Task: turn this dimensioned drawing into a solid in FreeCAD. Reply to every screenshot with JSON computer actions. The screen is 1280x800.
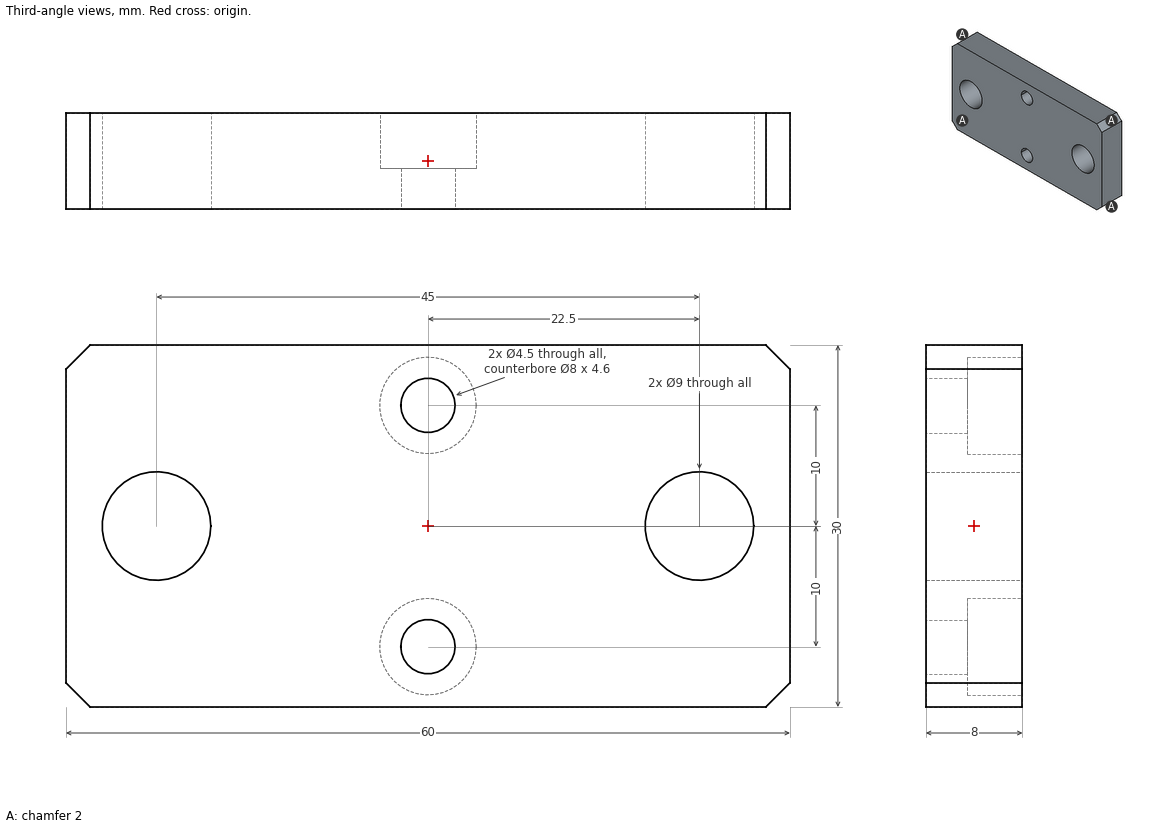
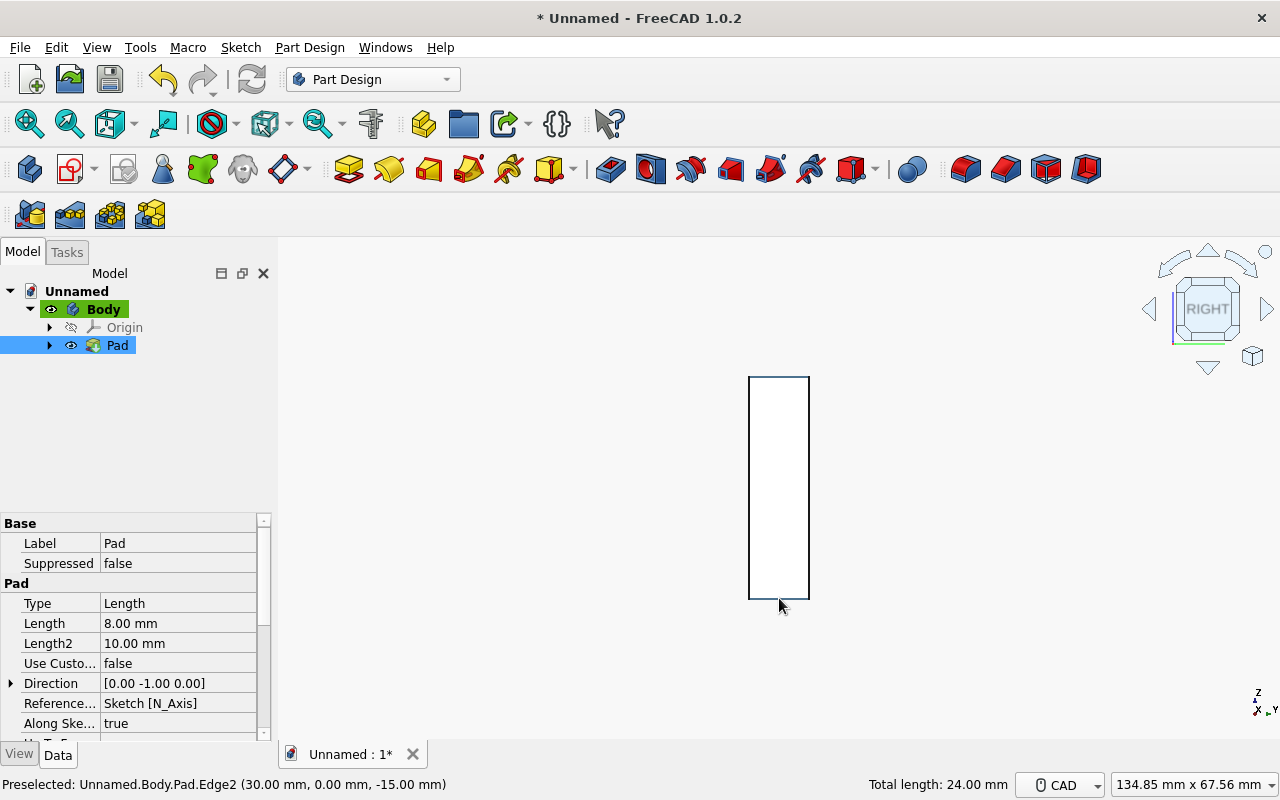
{"action": "key", "text": "5"}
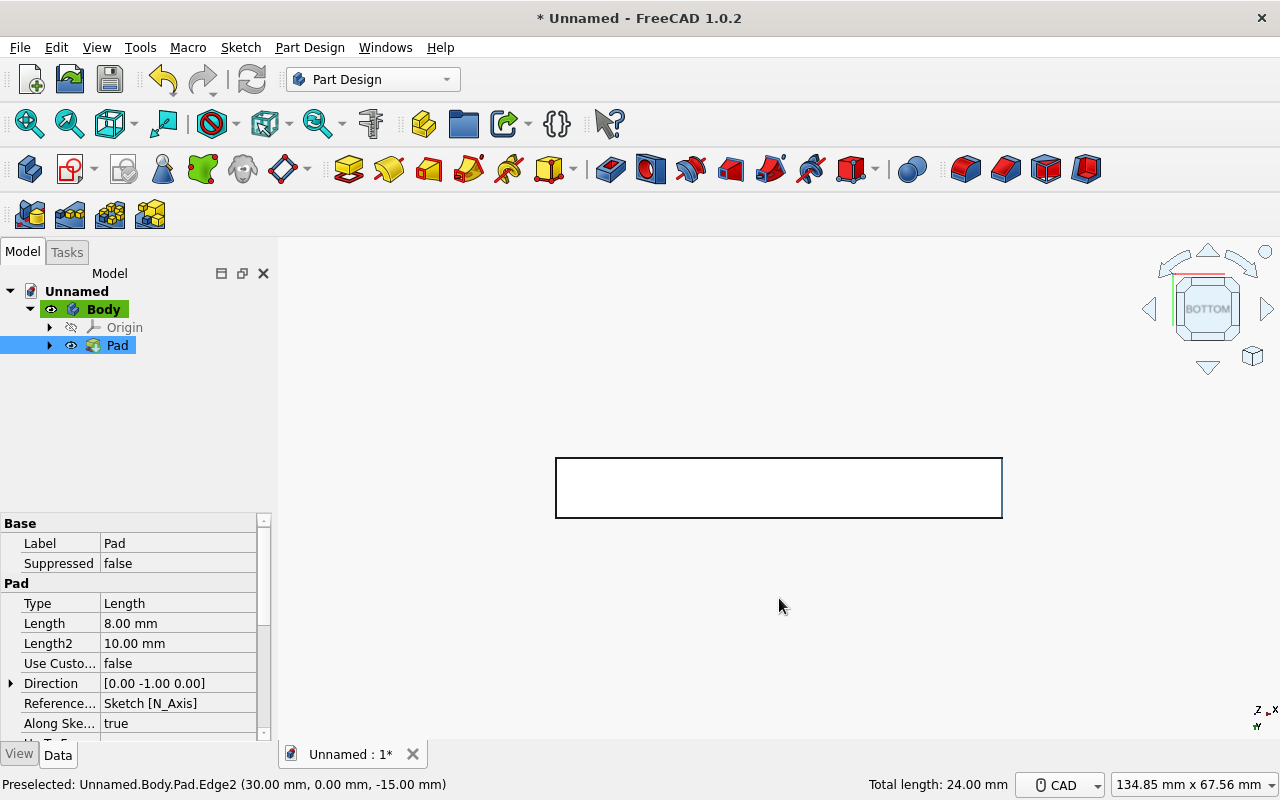
{"action": "left_click", "coordinate": [30, 124]}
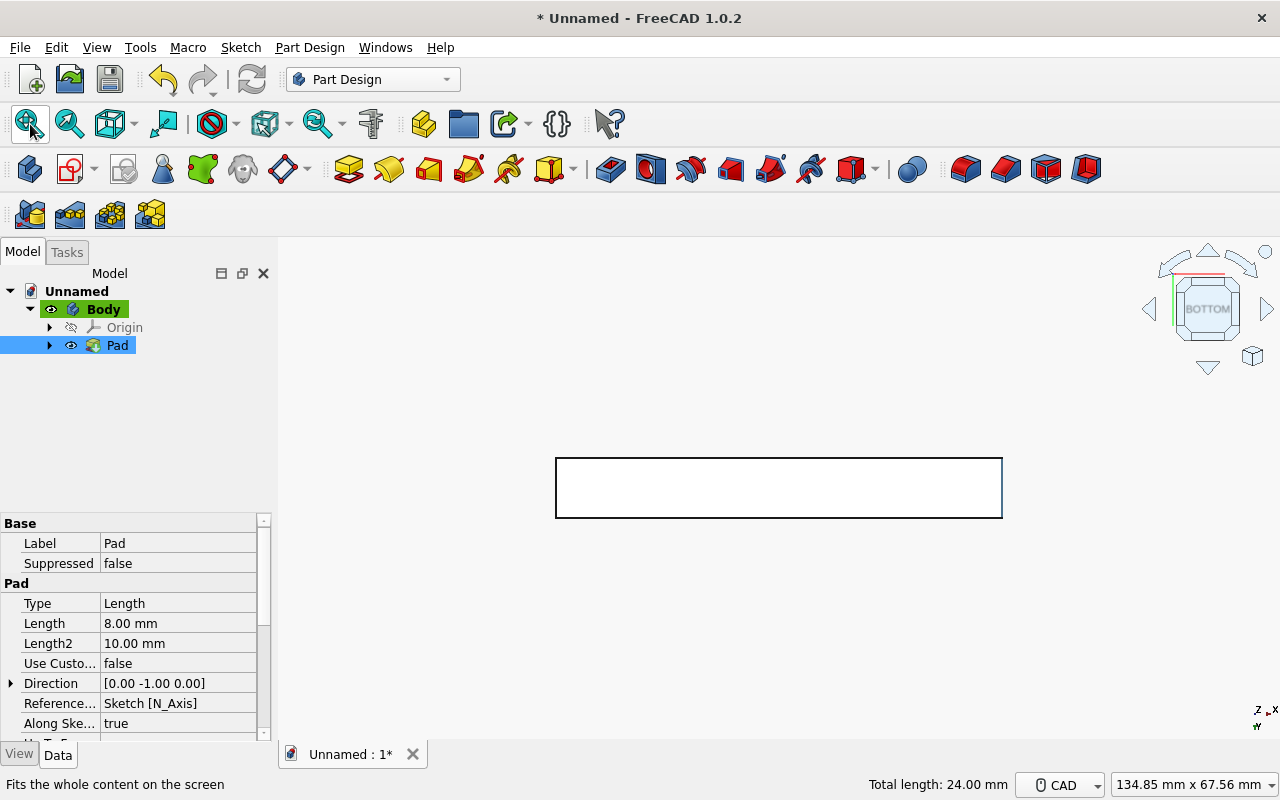
{"action": "left_click", "coordinate": [556, 487], "text": "ctrl"}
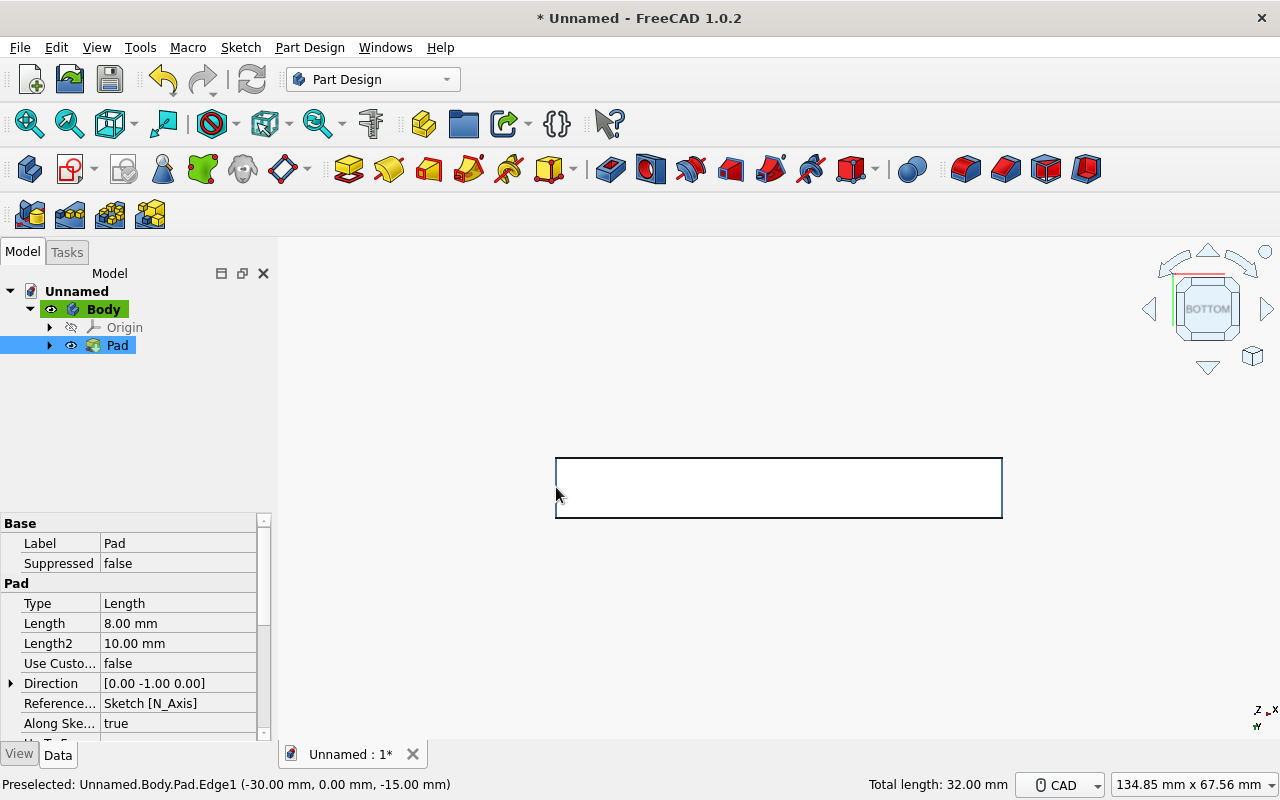
{"action": "left_click", "coordinate": [1006, 170]}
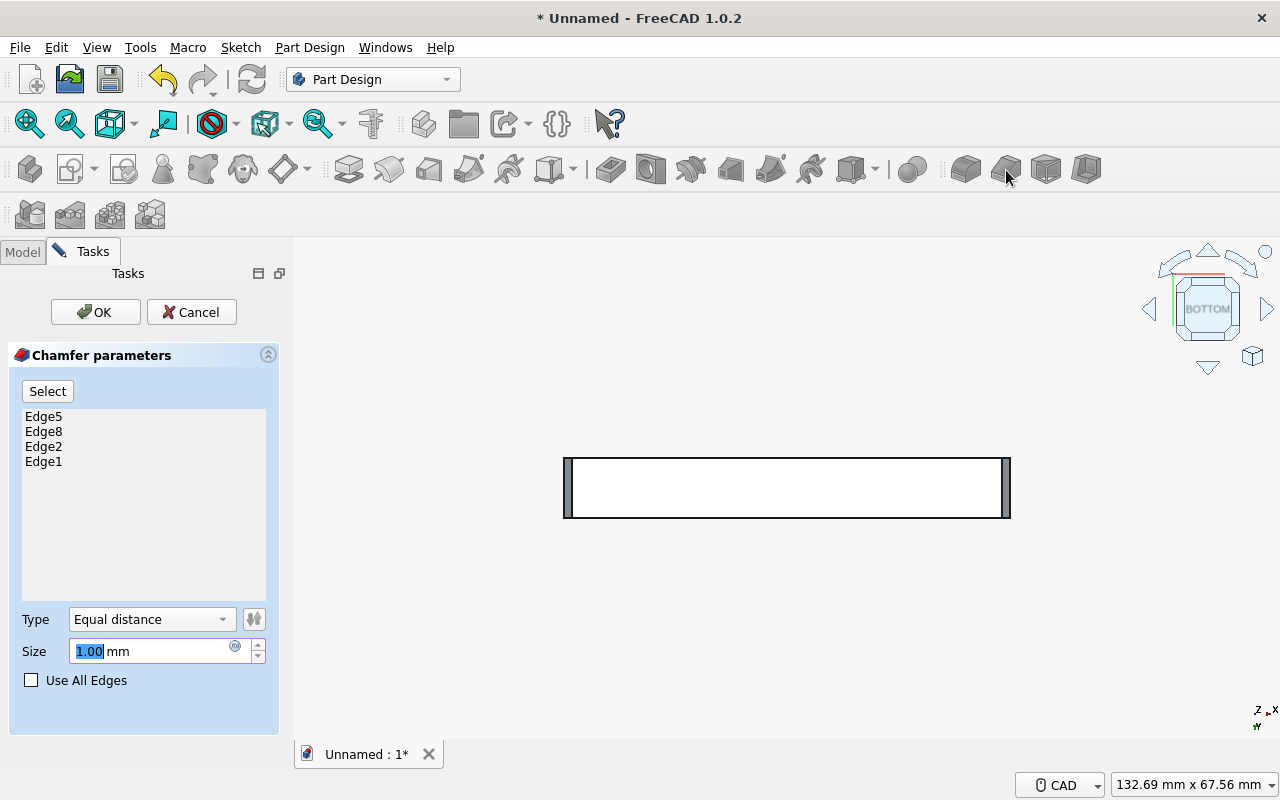
{"action": "type", "text": "2"}
{"action": "key", "text": "Tab"}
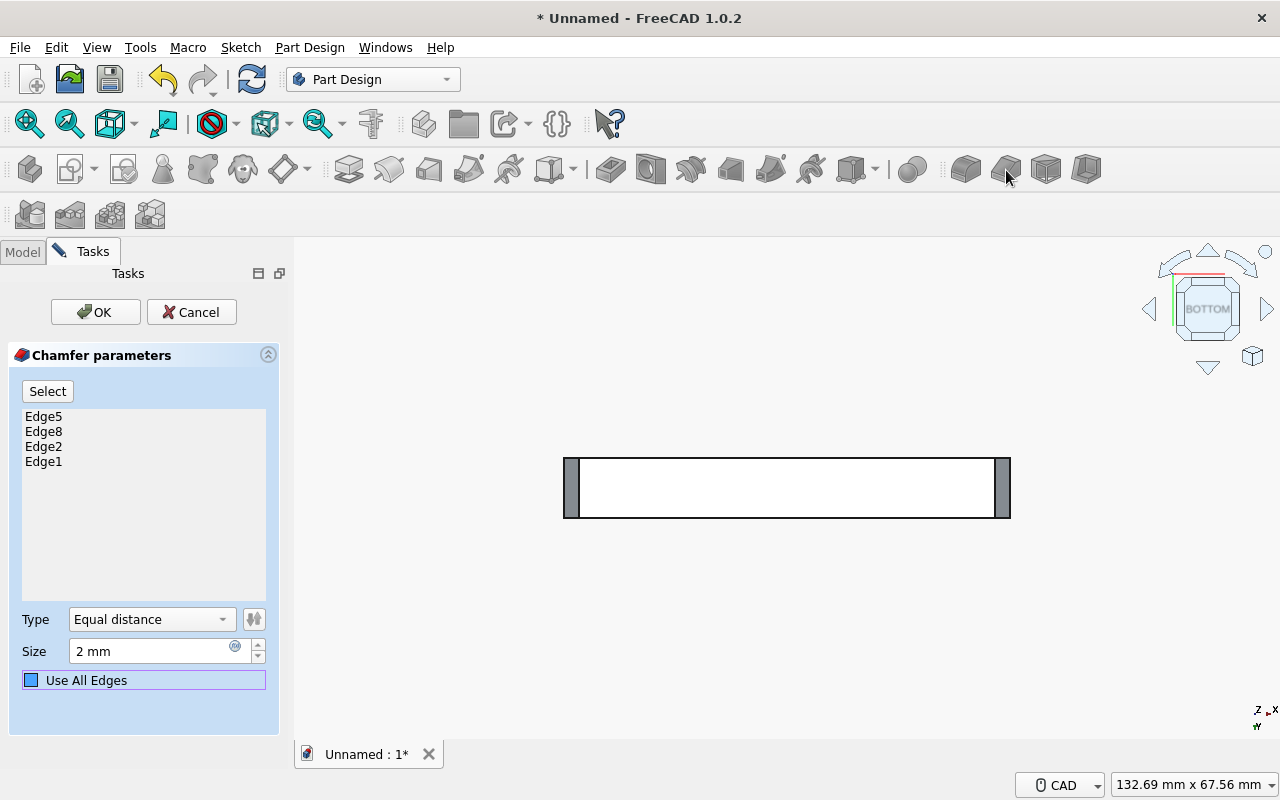
{"action": "left_click", "coordinate": [96, 312]}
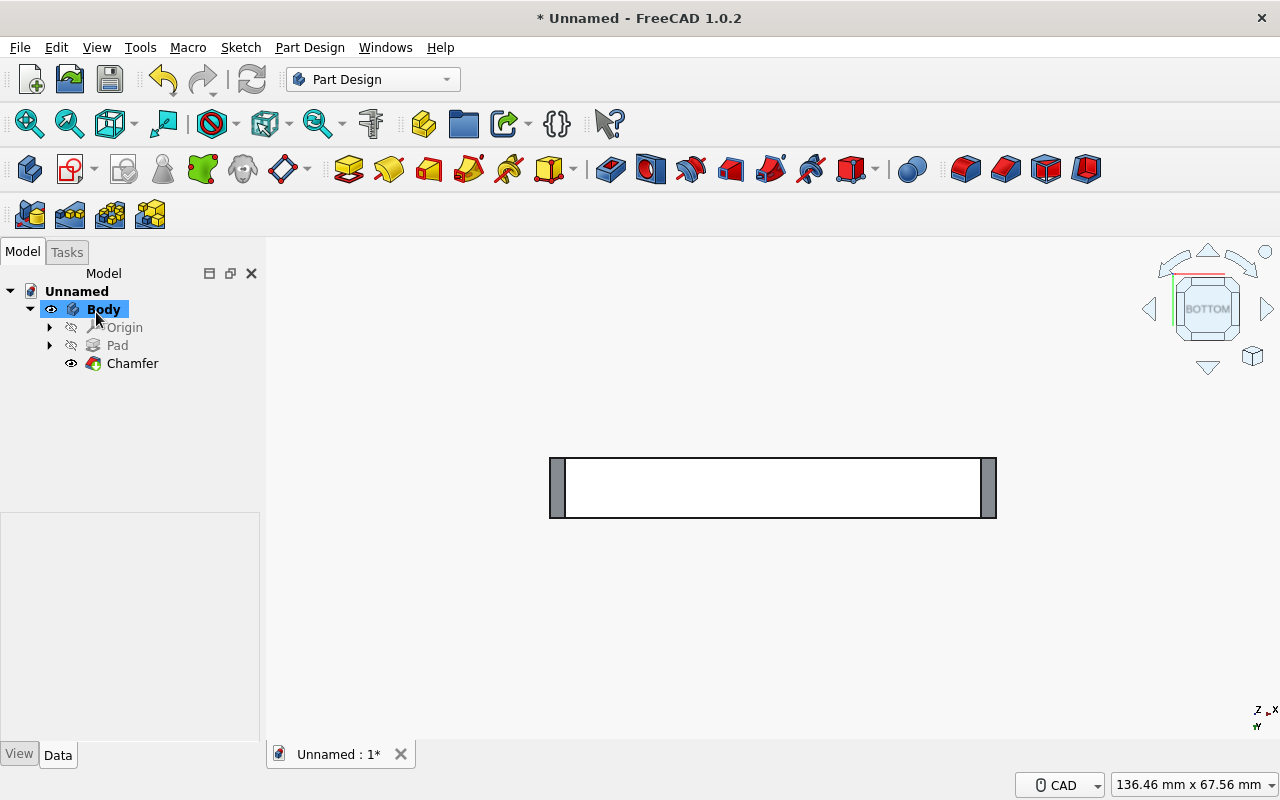
{"action": "left_click", "coordinate": [30, 124]}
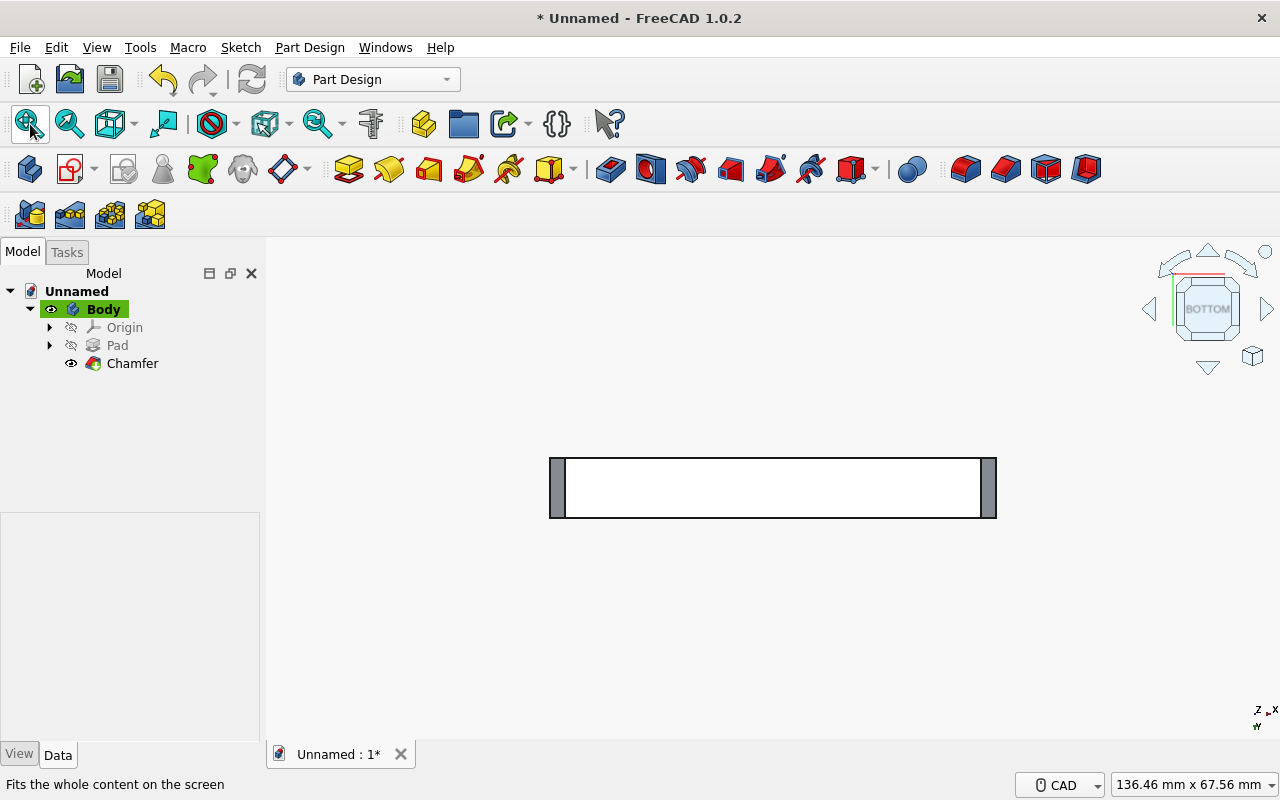
{"action": "key", "text": "4"}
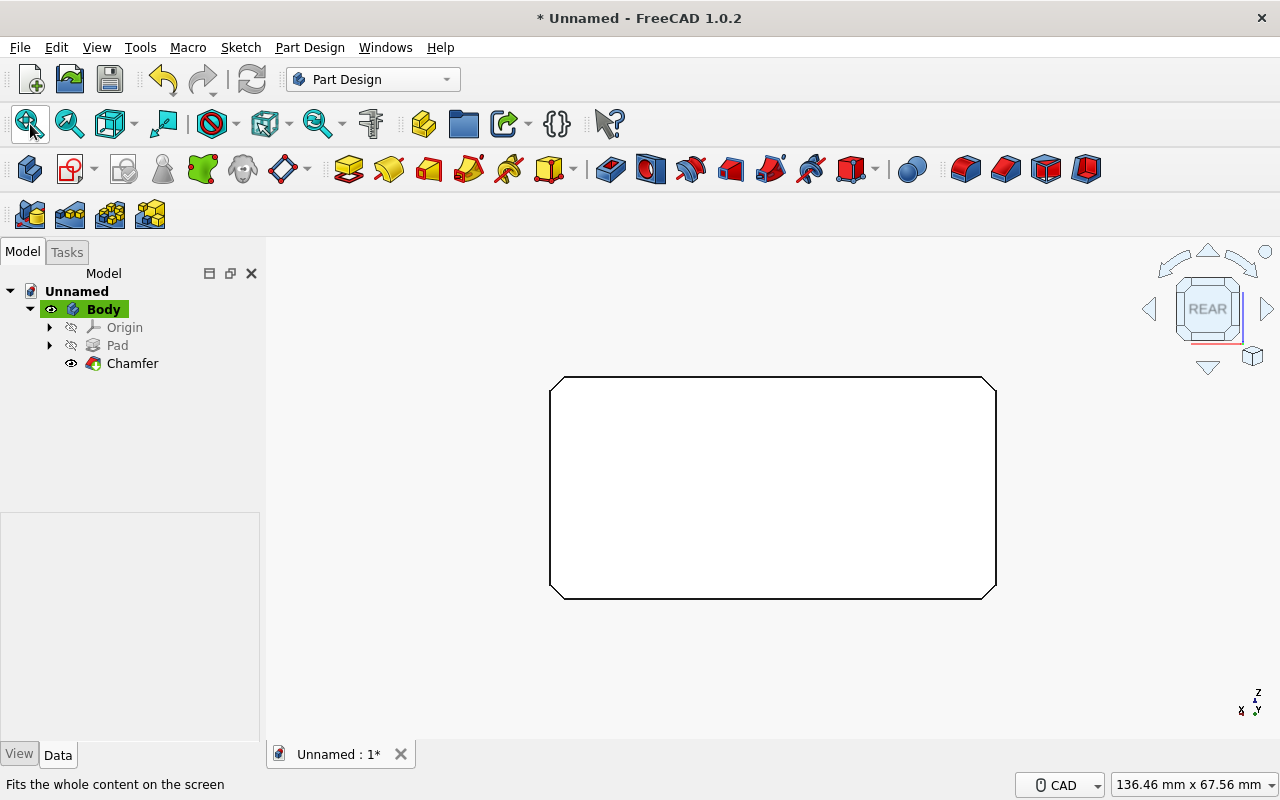
{"action": "left_click", "coordinate": [30, 124]}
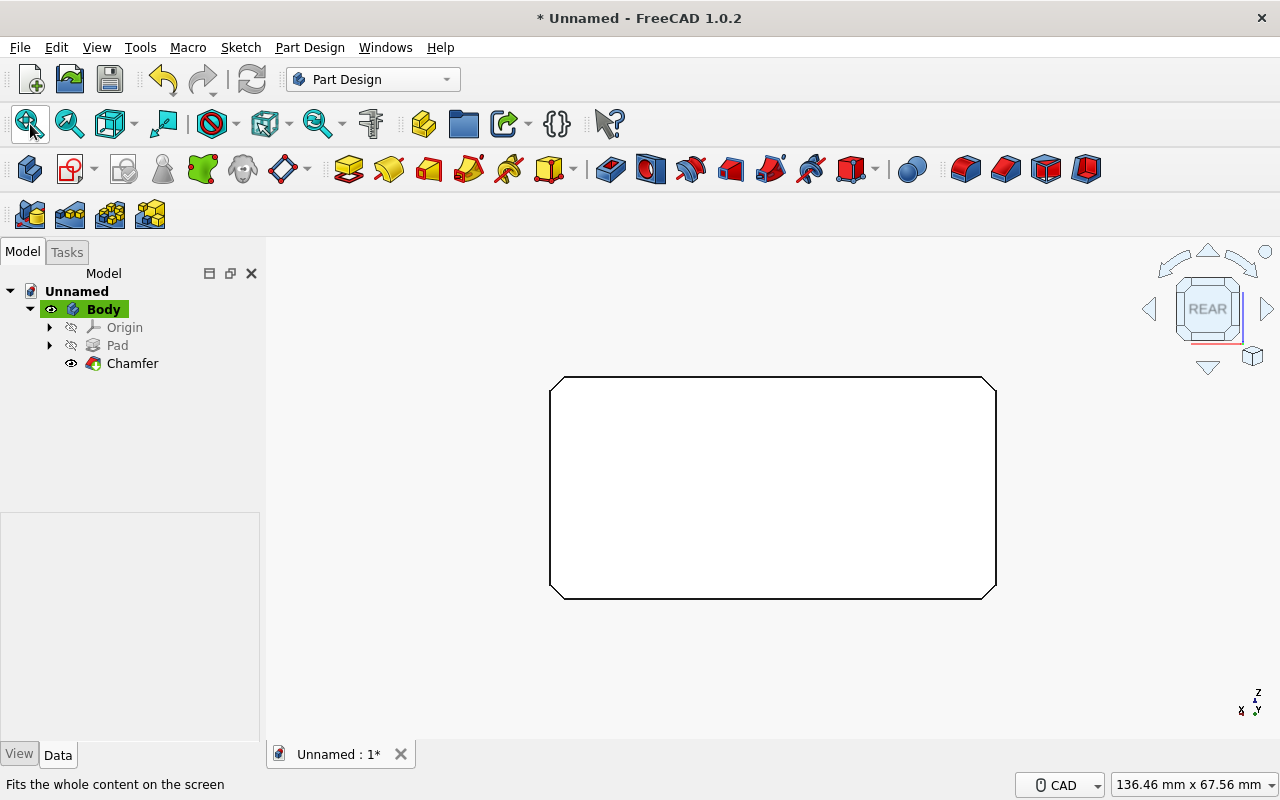
{"action": "left_click", "coordinate": [709, 487]}